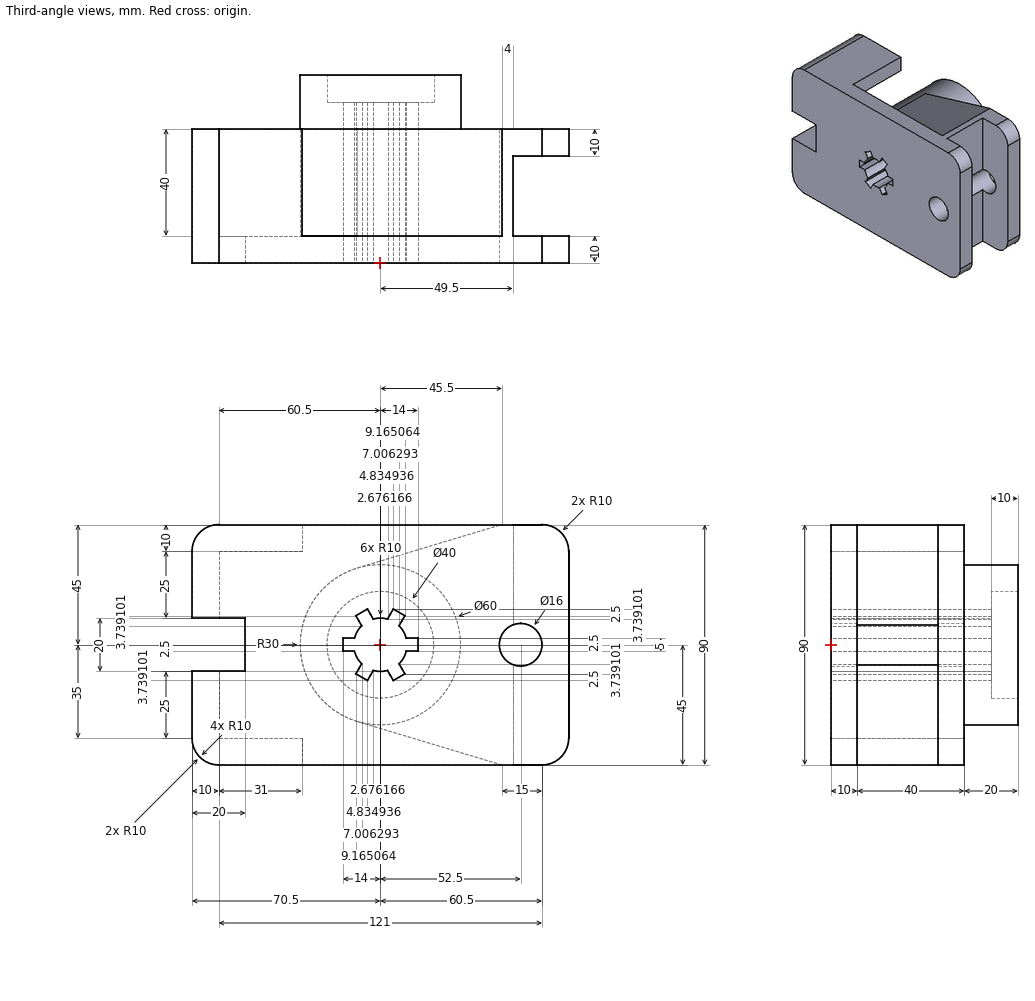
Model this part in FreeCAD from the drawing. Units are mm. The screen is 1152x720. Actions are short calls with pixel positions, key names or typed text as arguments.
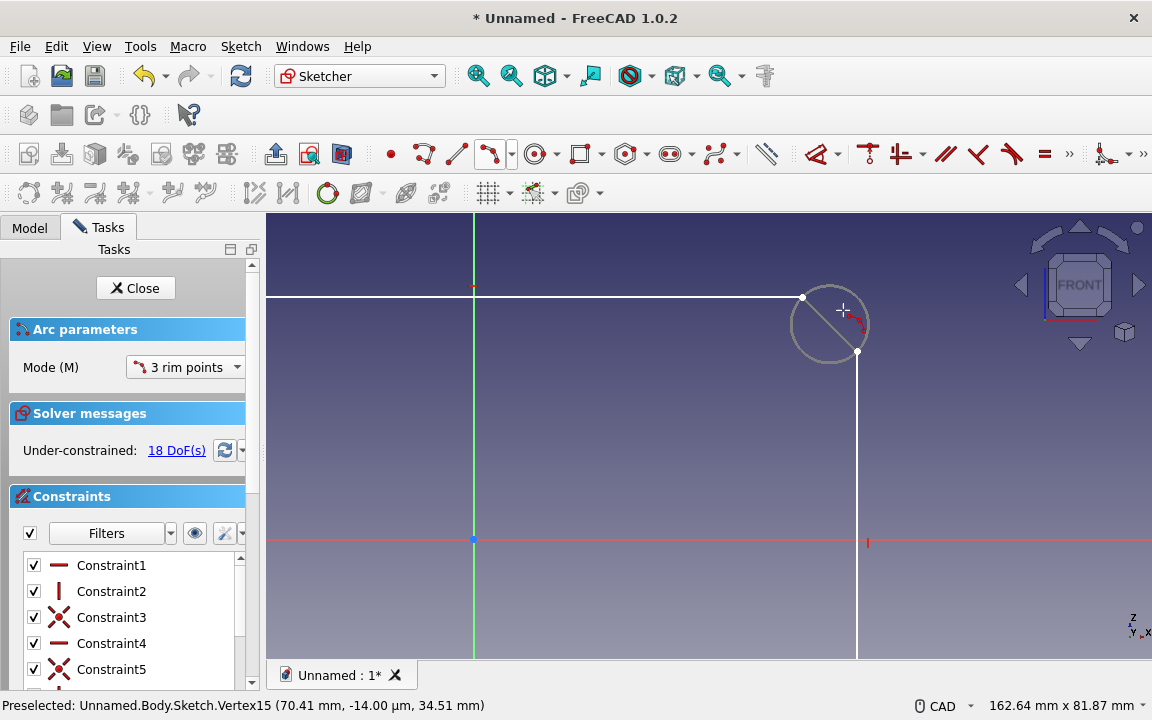
click(842, 311)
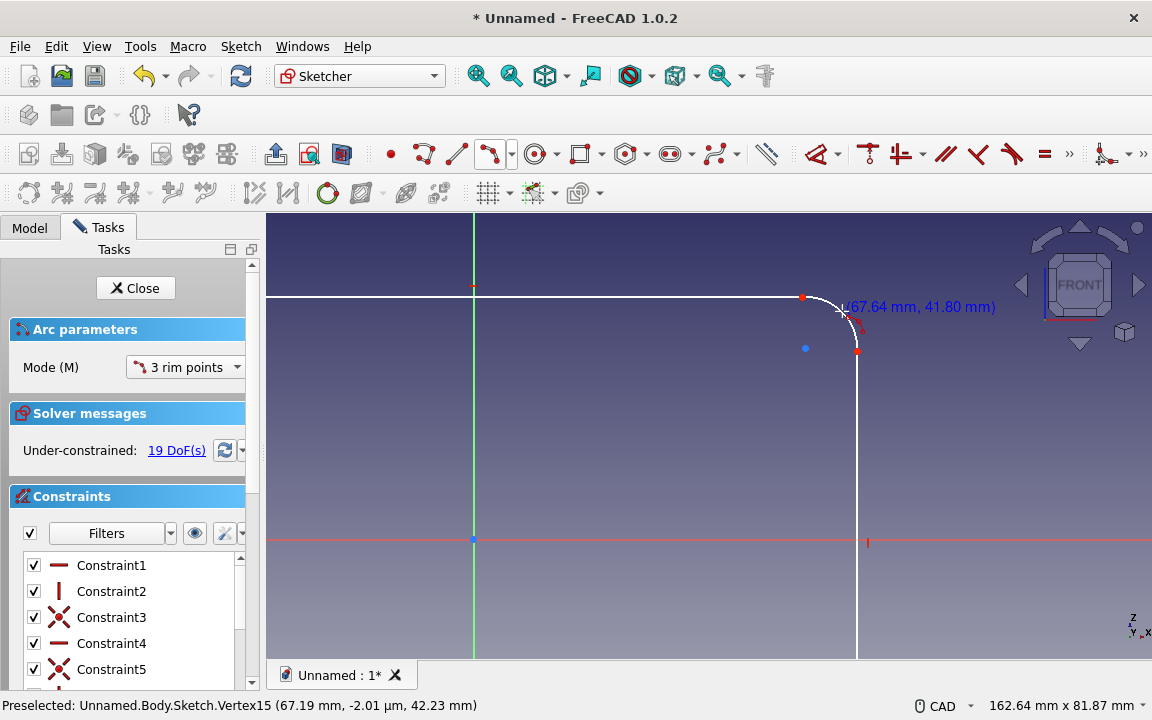
scroll(844, 310, down, 3)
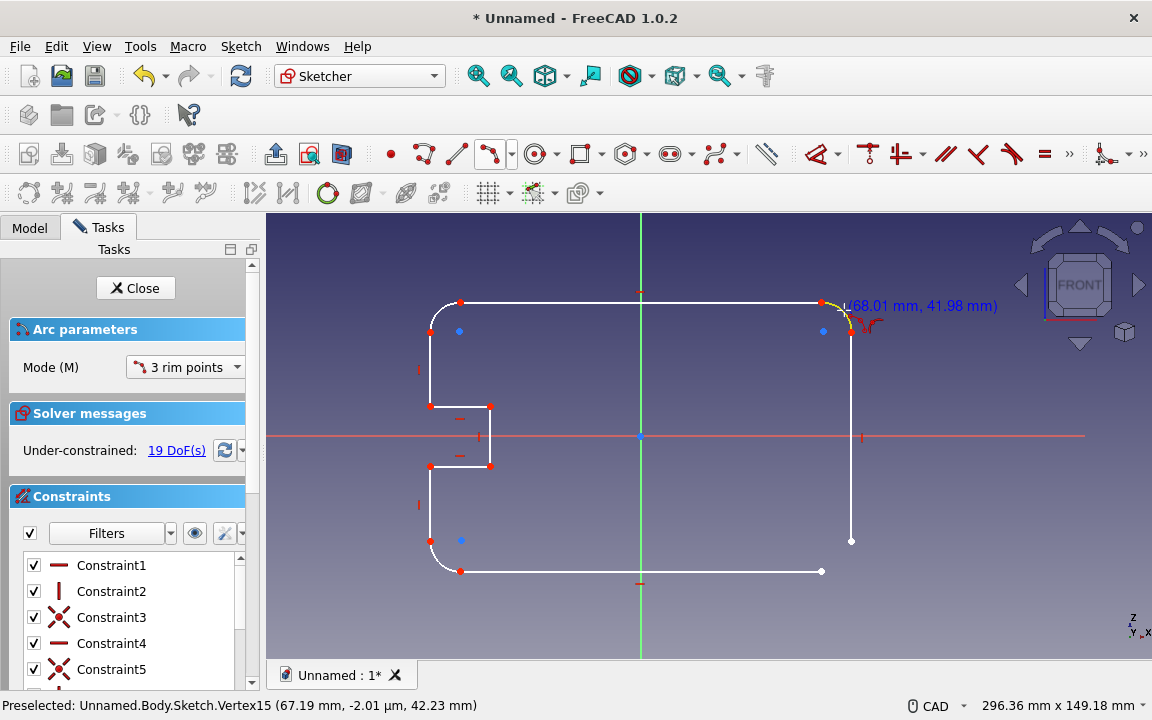
click(851, 542)
click(821, 572)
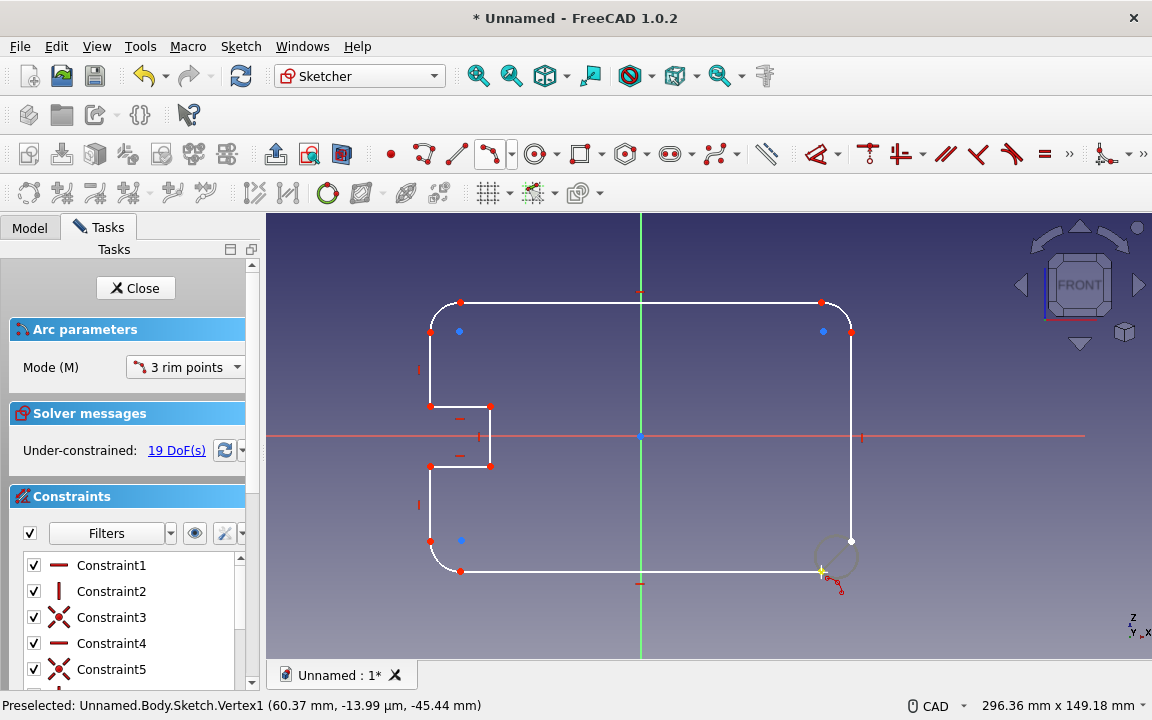
scroll(843, 562, up, 3)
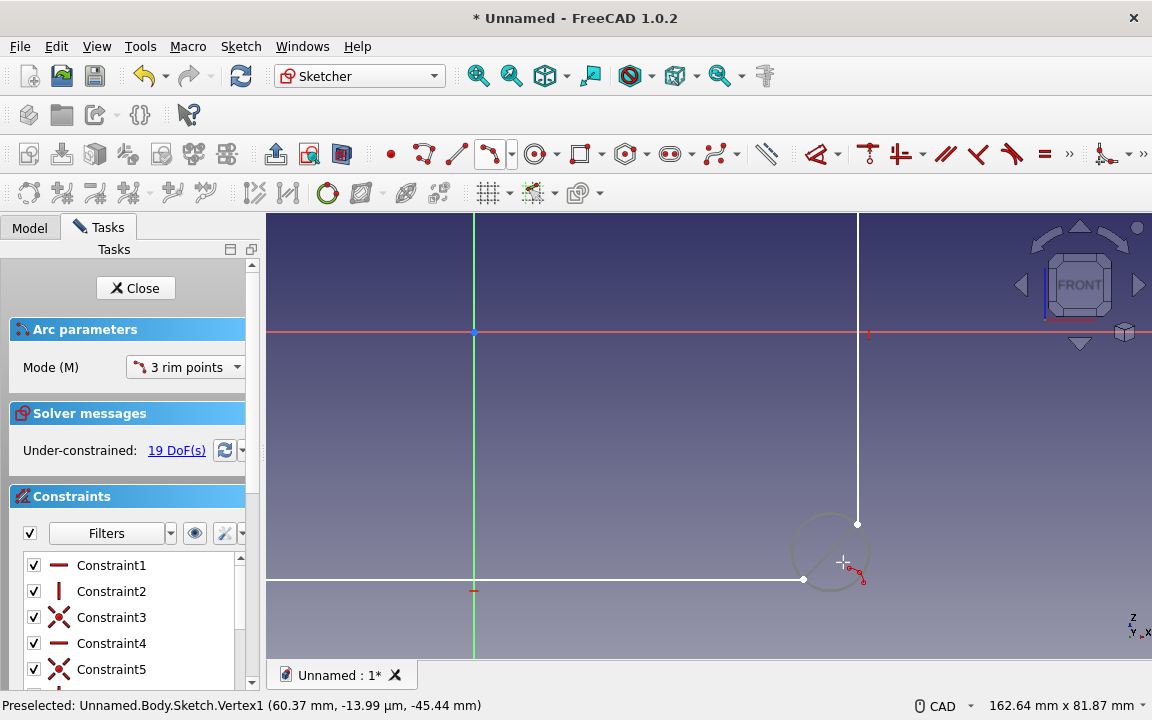
click(842, 561)
key(Escape)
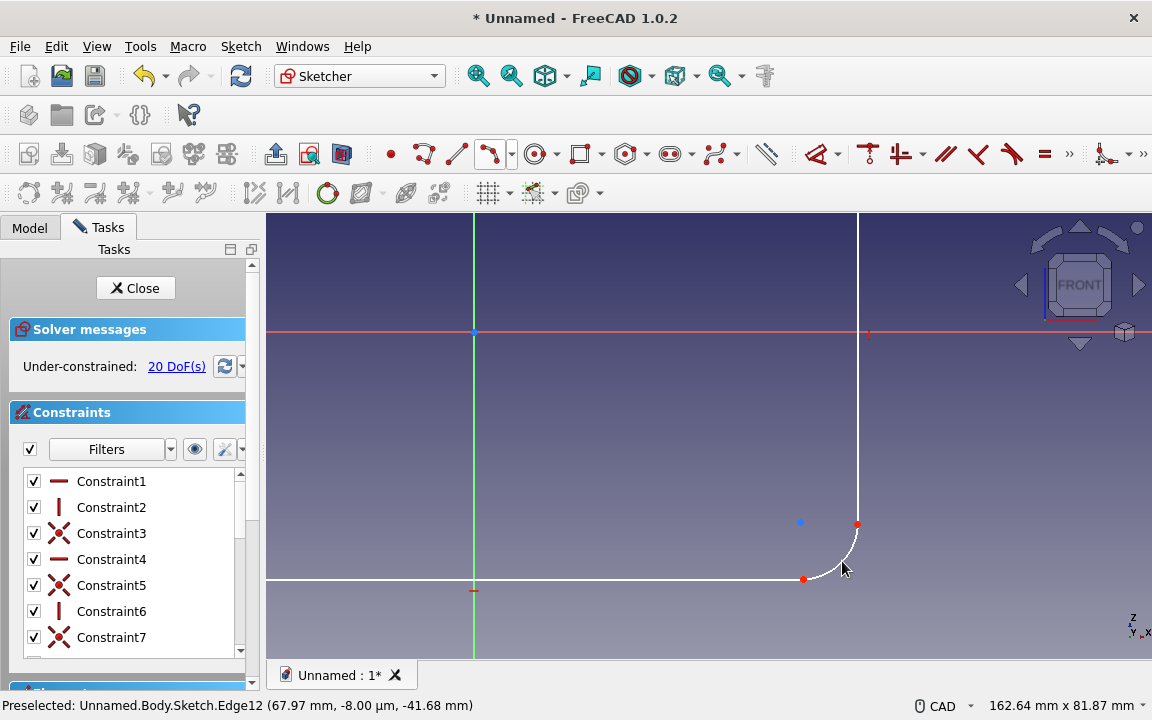
click(606, 580)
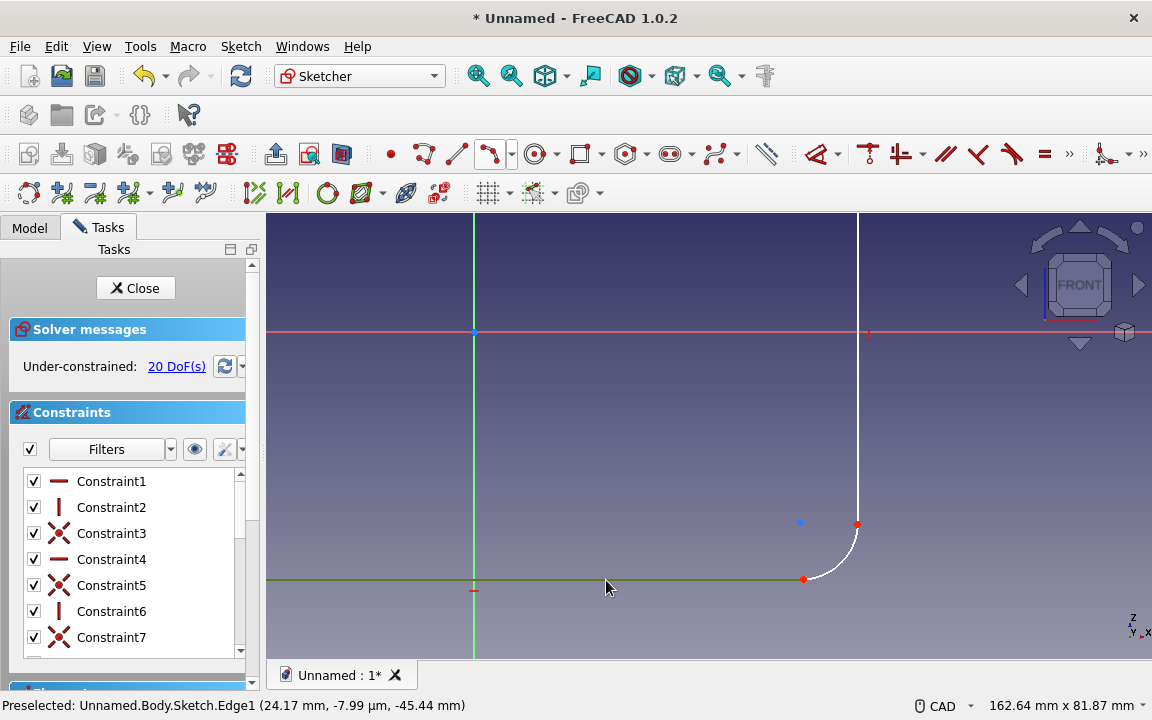
scroll(843, 562, down, 3)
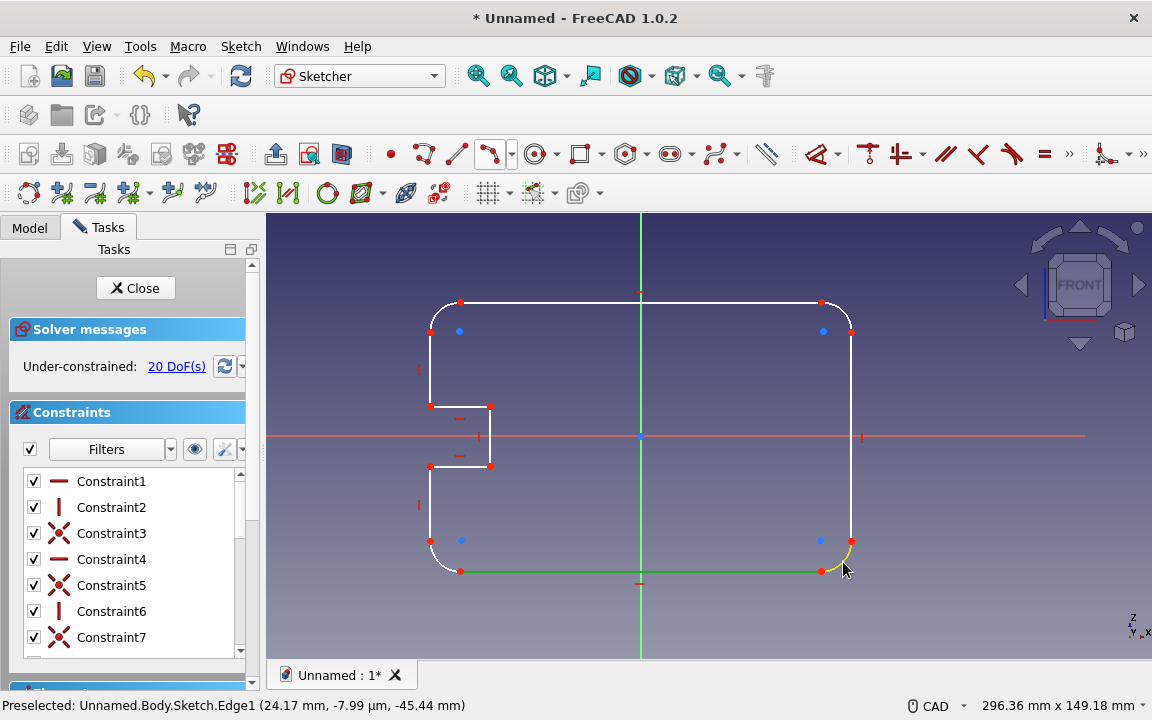
click(434, 555)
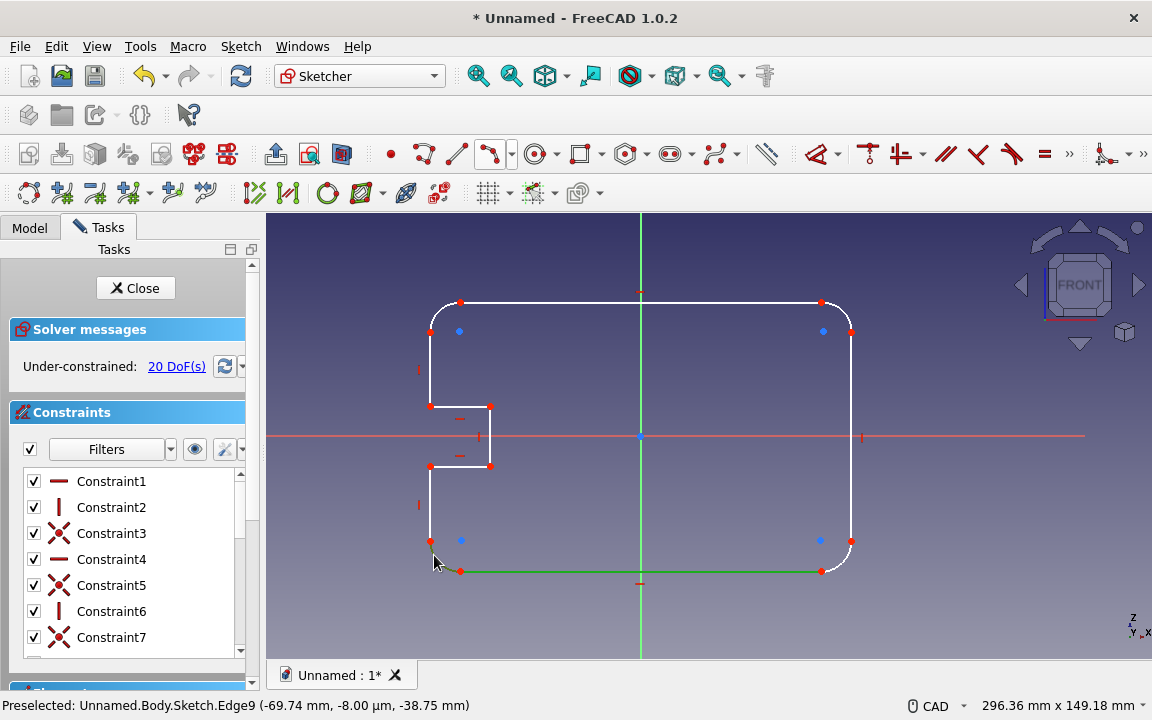
click(1012, 154)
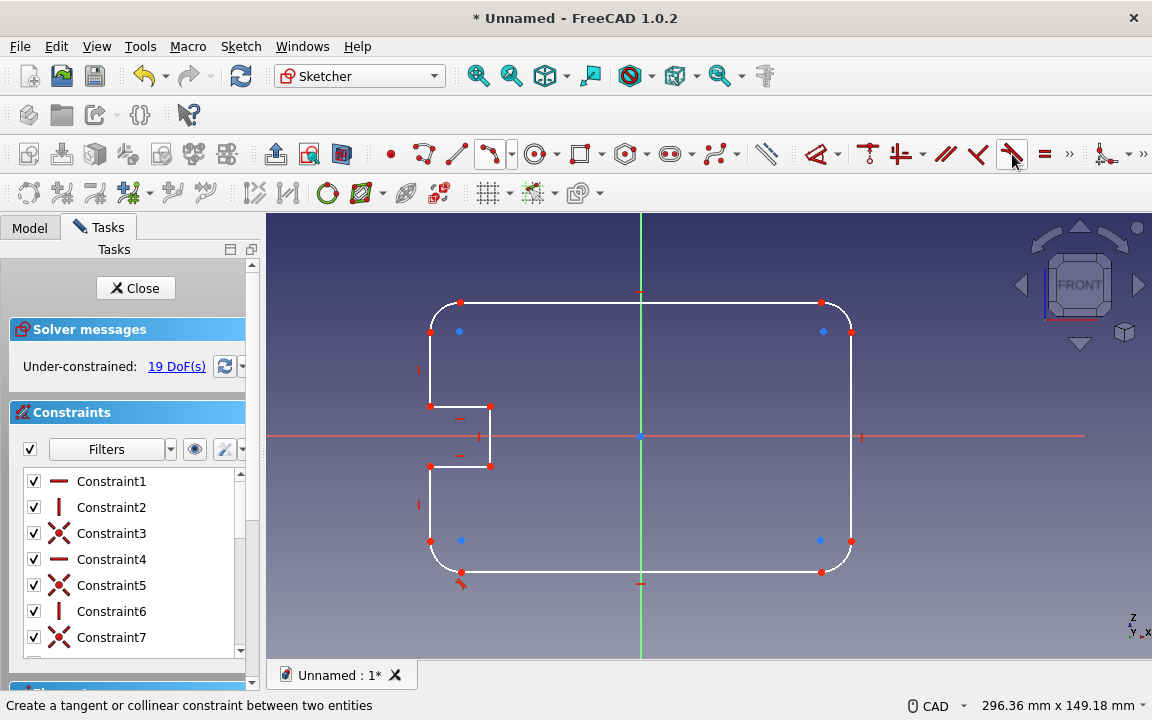
click(713, 572)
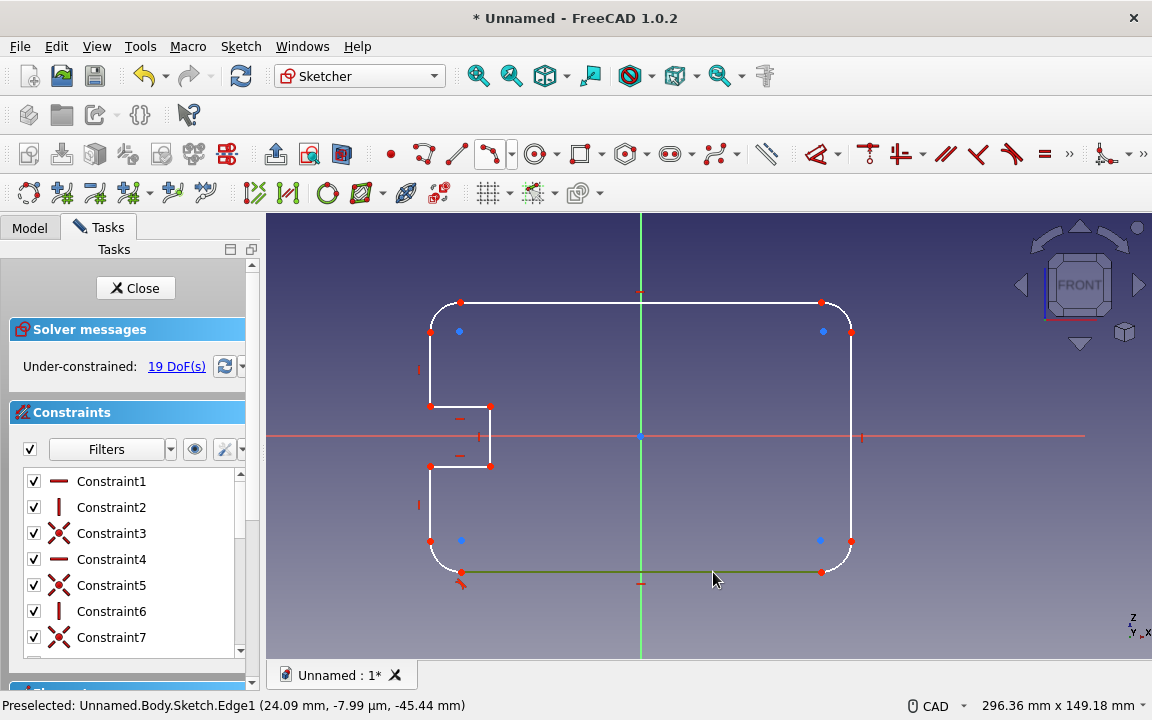
click(835, 568)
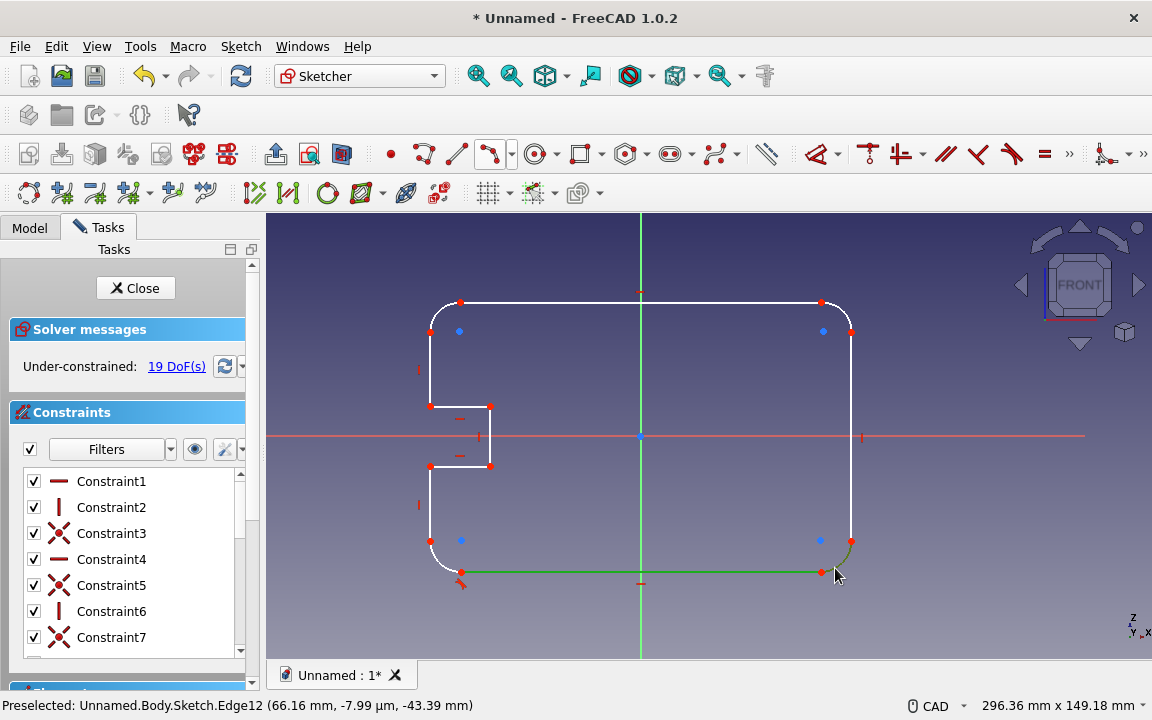
click(1012, 154)